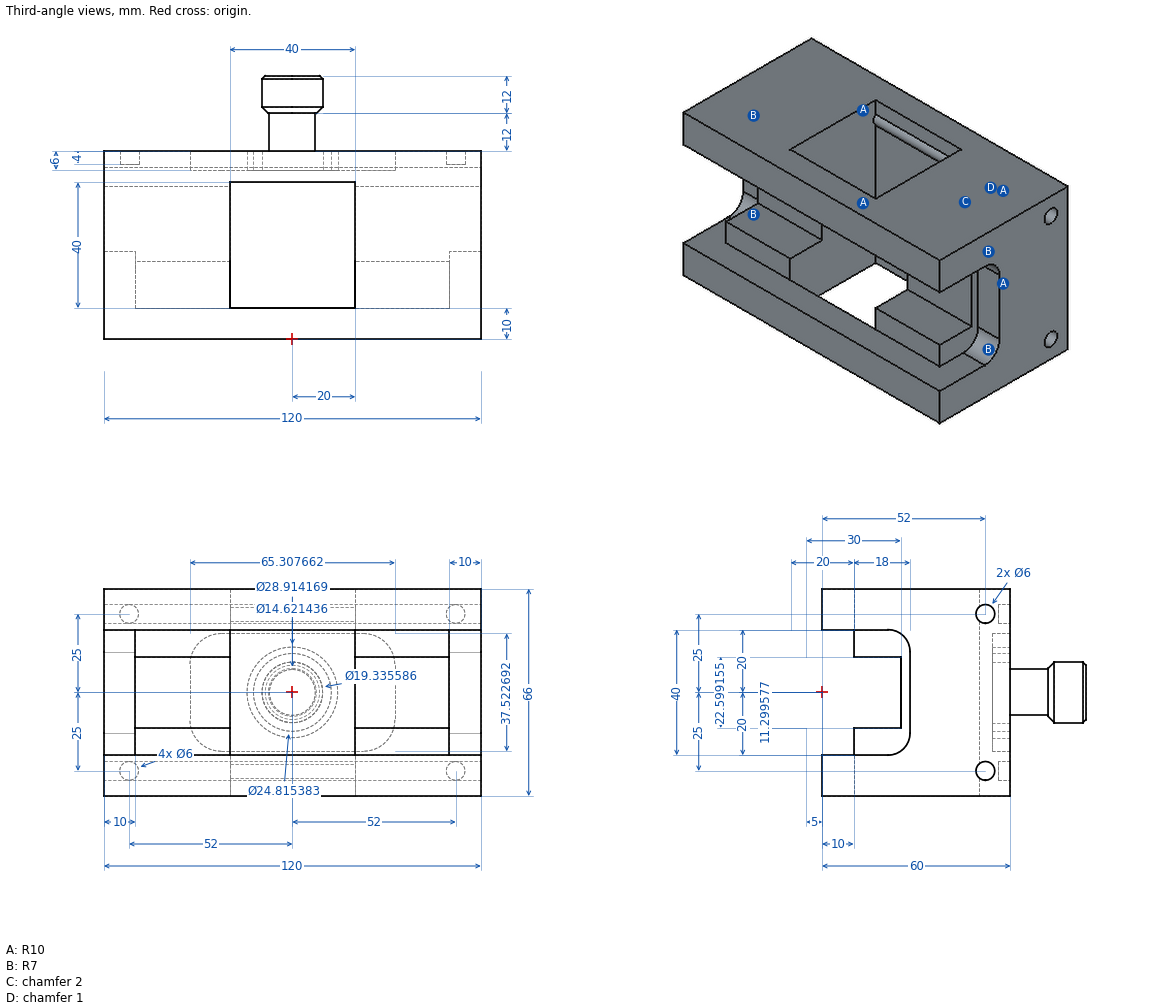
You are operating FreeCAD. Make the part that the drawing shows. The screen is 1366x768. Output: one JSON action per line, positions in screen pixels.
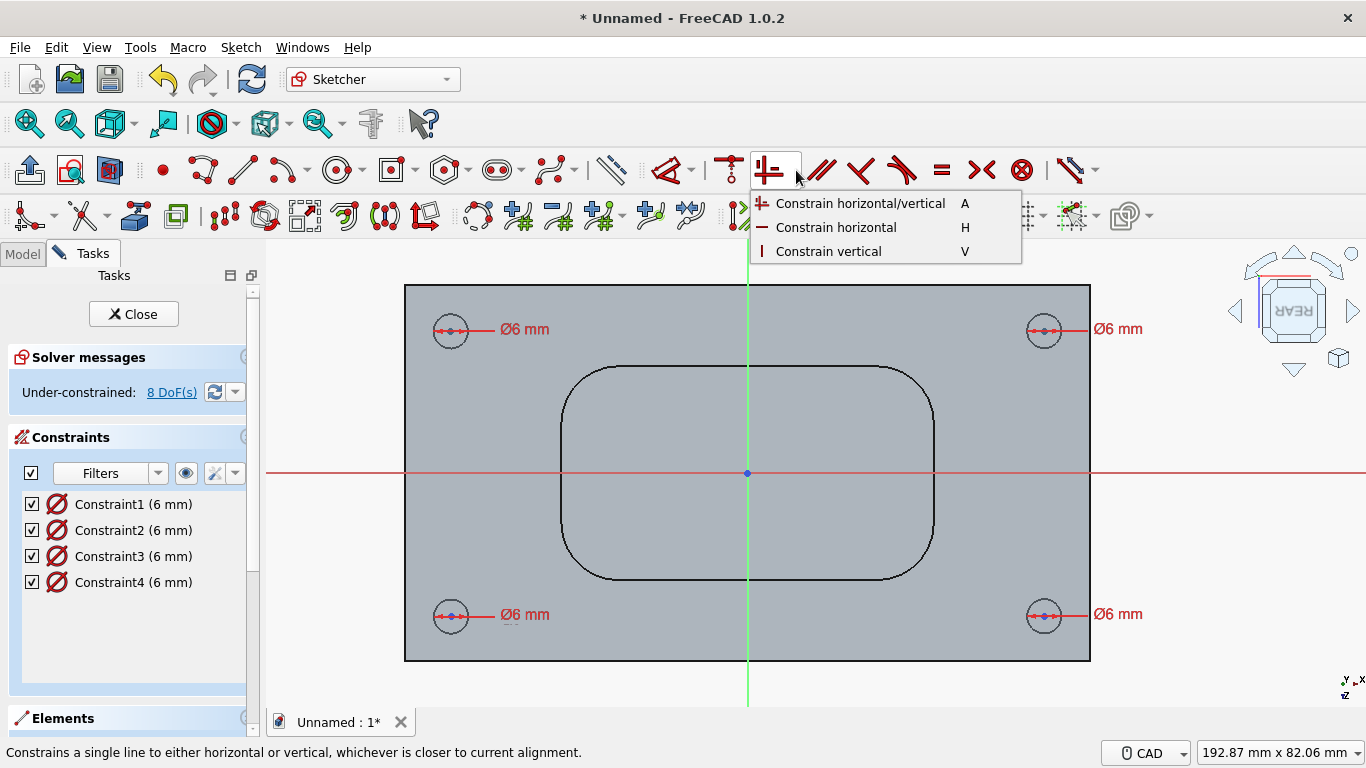
{"action": "left_click", "coordinate": [886, 227]}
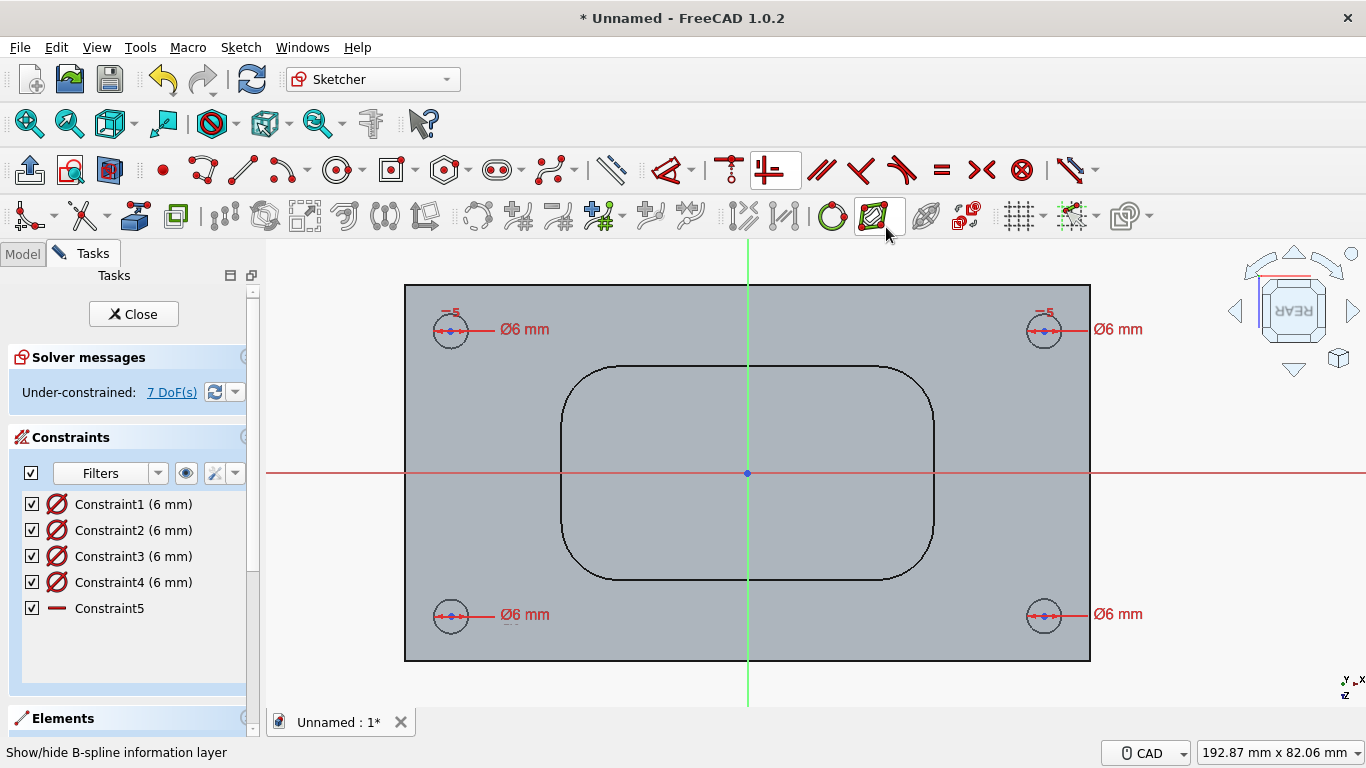
{"action": "left_click", "coordinate": [451, 331]}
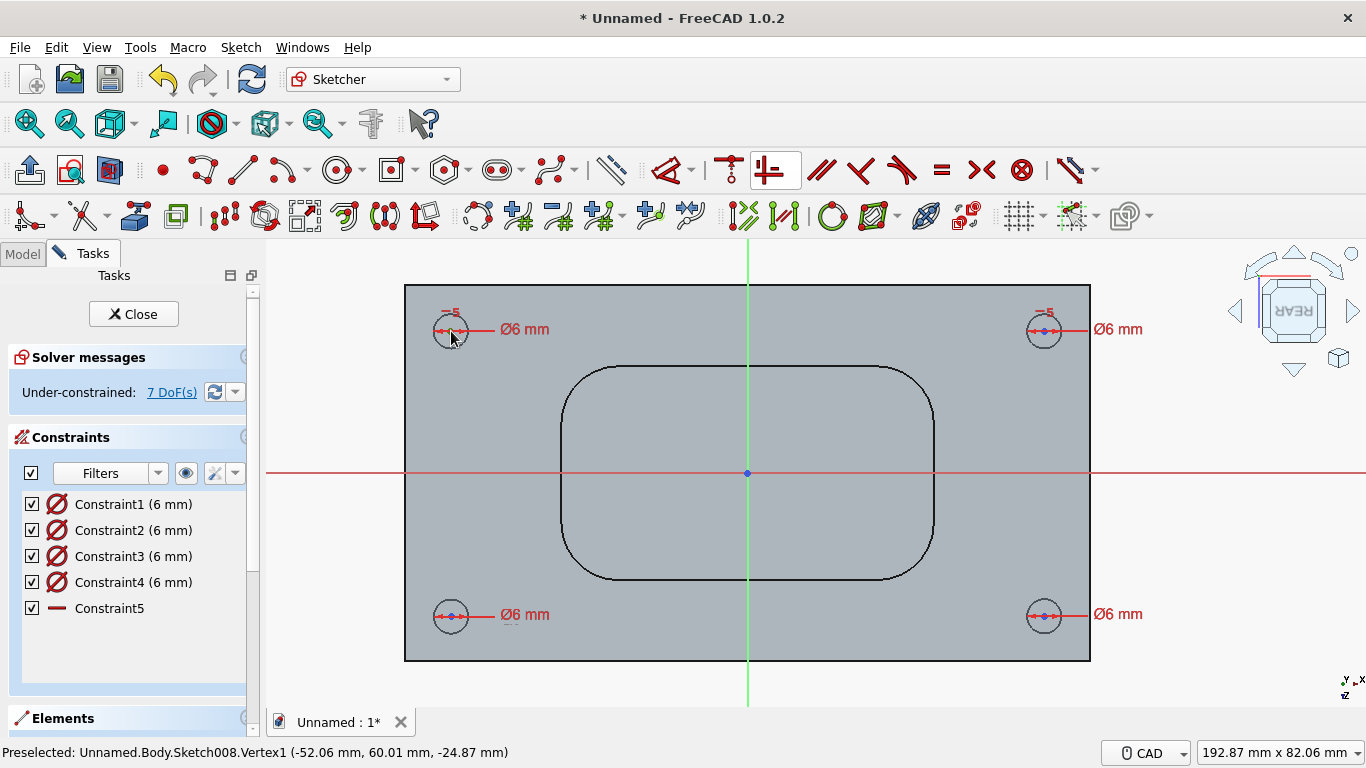
{"action": "left_click", "coordinate": [451, 617]}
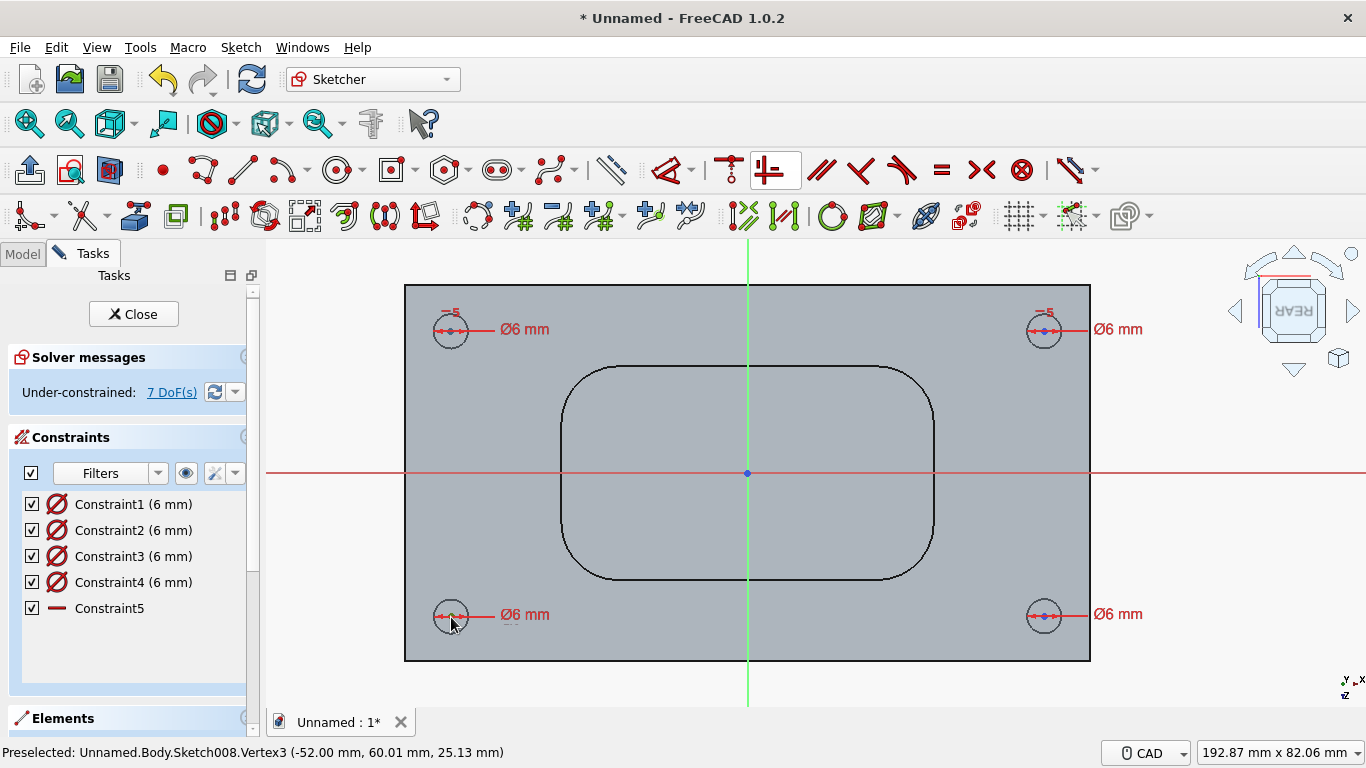
{"action": "left_click", "coordinate": [796, 170]}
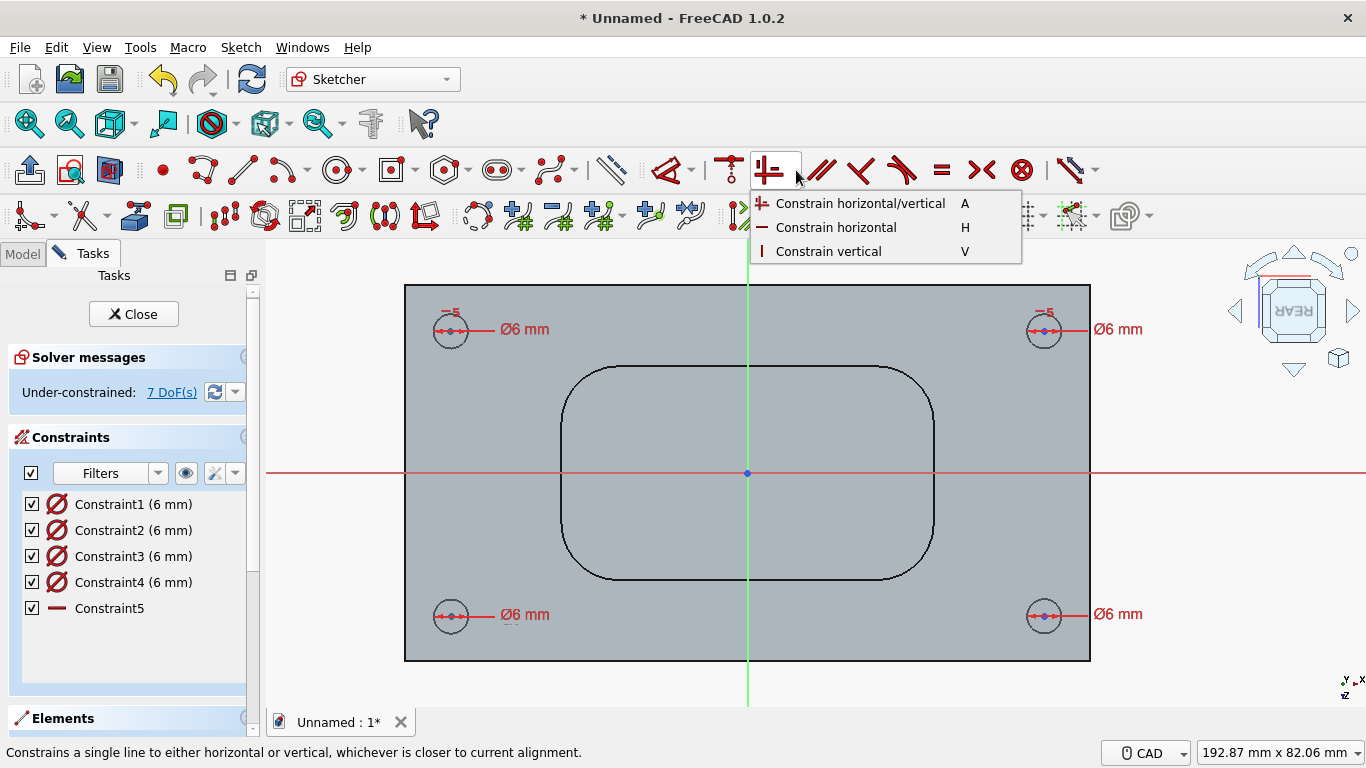
{"action": "left_click", "coordinate": [886, 251]}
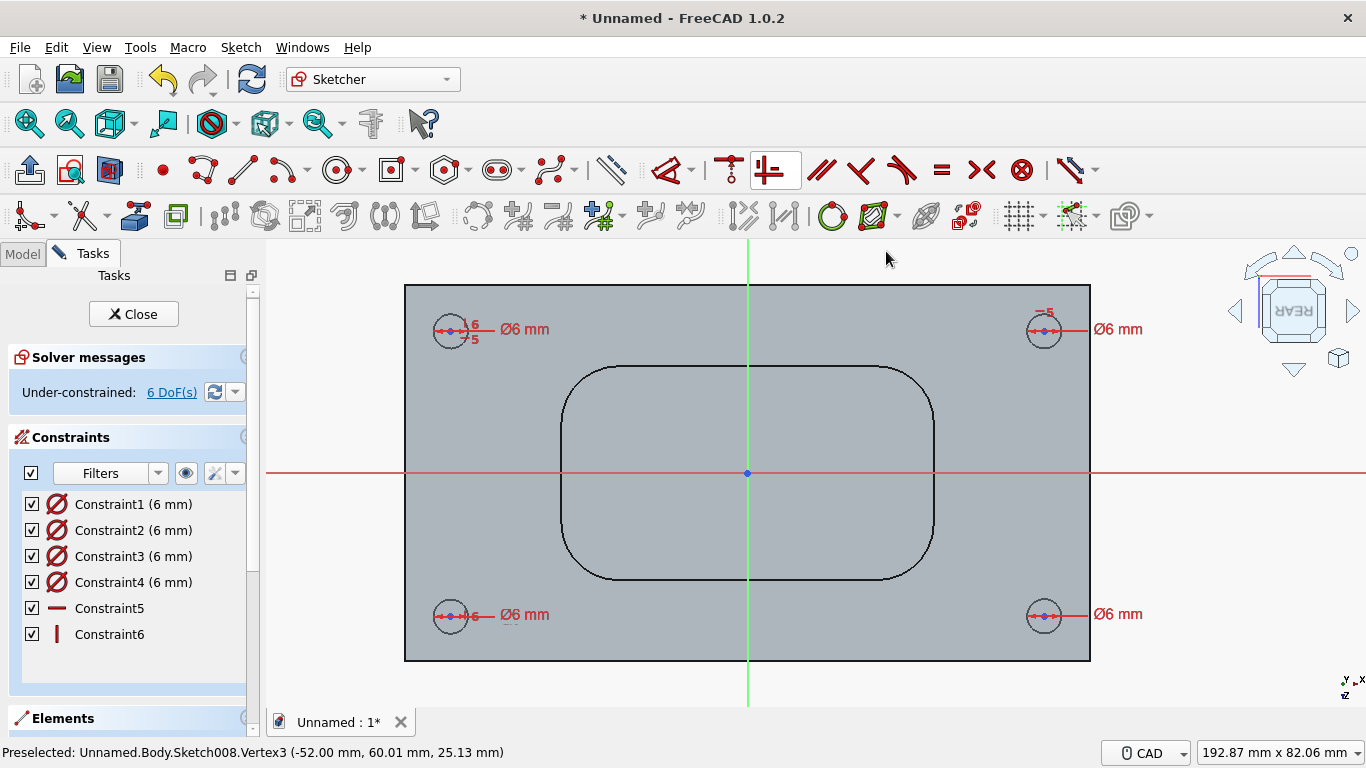
{"action": "left_click", "coordinate": [1044, 331]}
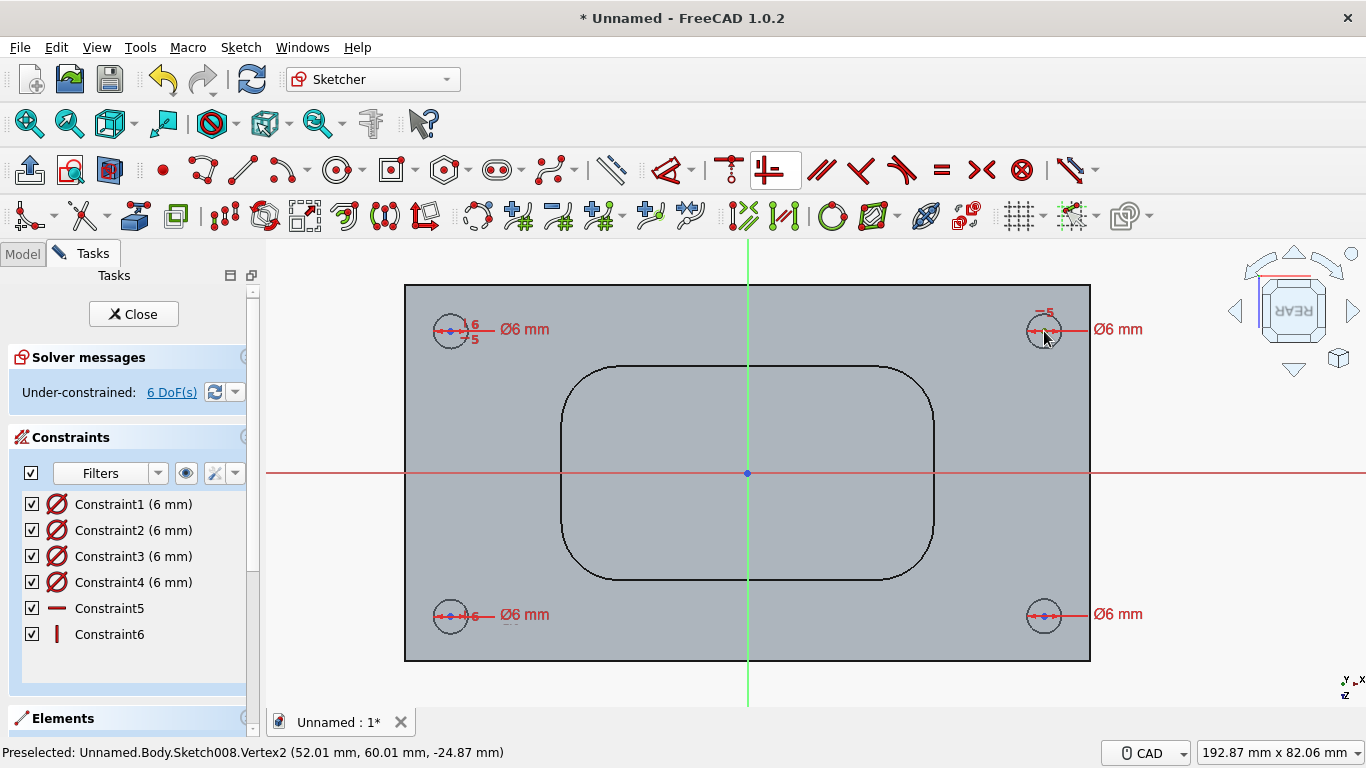
{"action": "left_click", "coordinate": [1044, 616]}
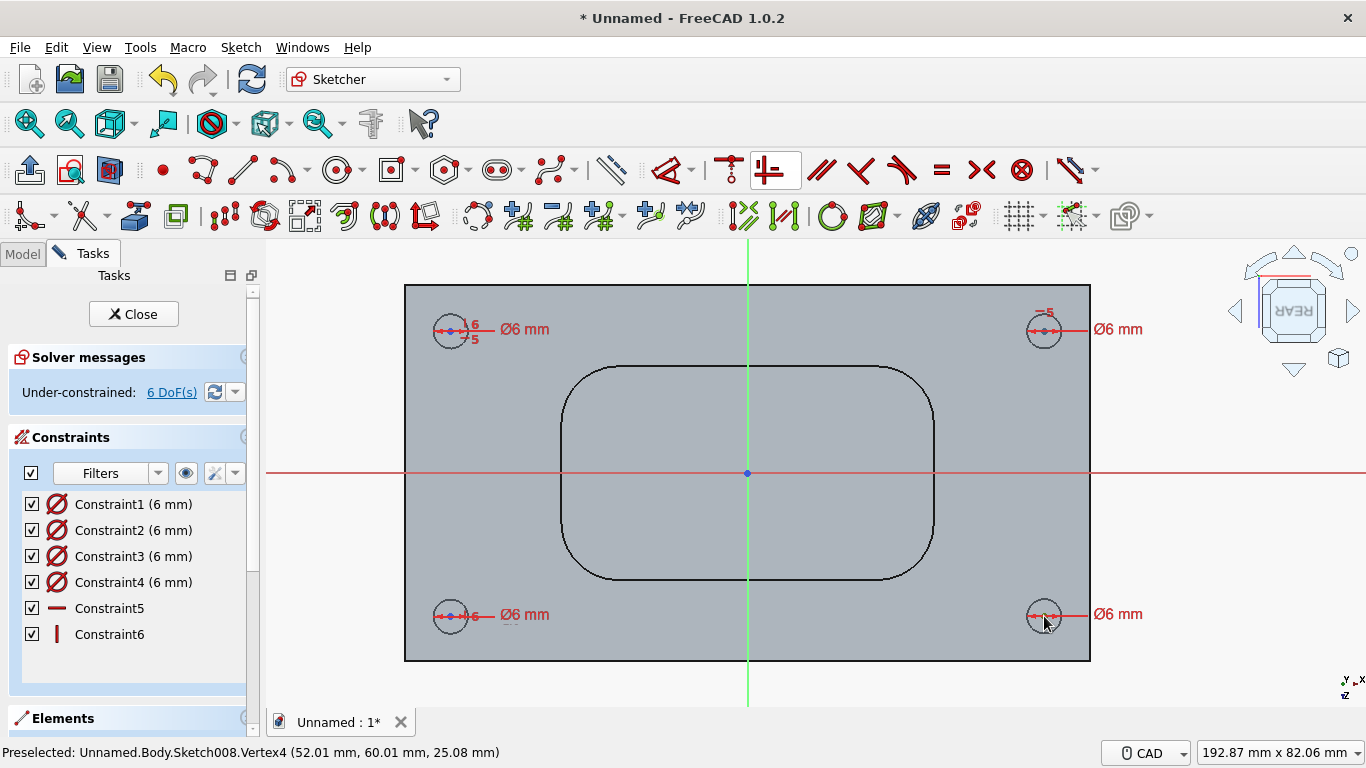
{"action": "left_click", "coordinate": [796, 170]}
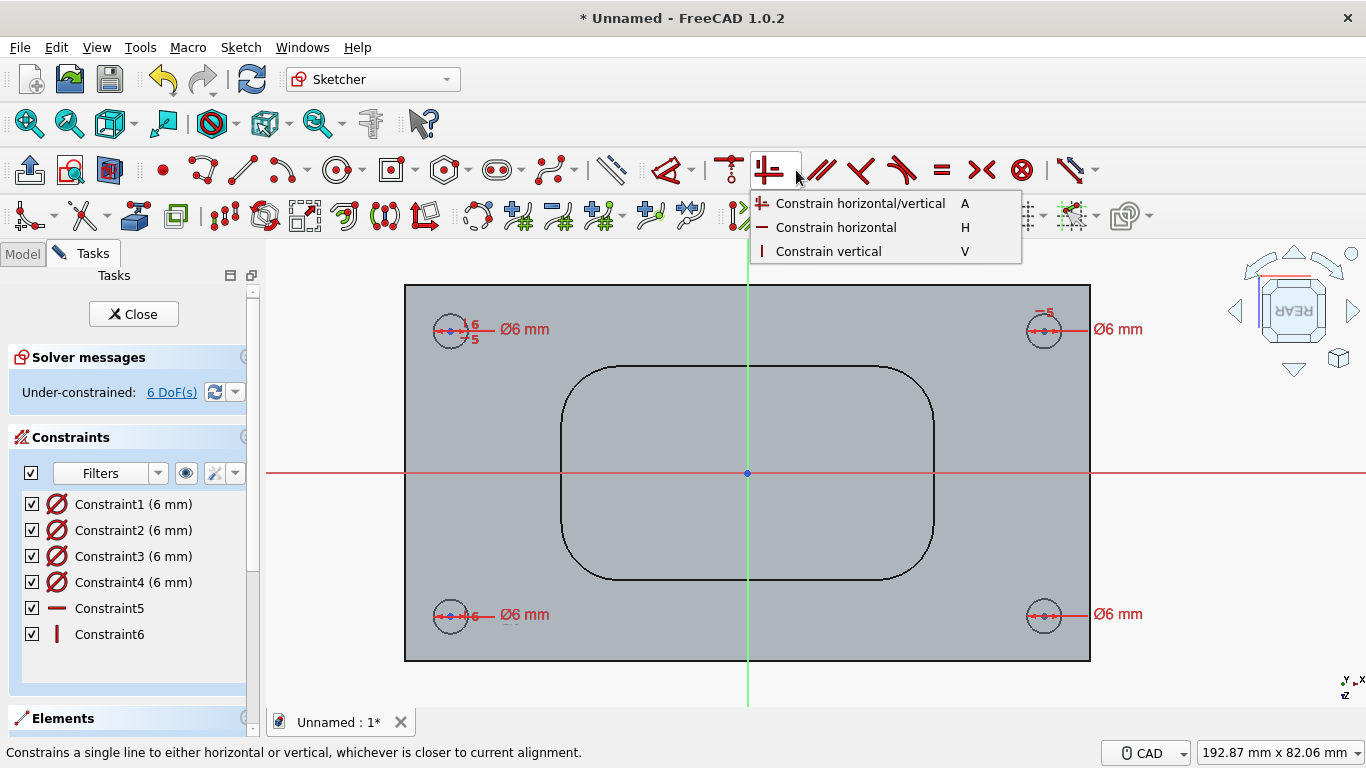
{"action": "left_click", "coordinate": [886, 251]}